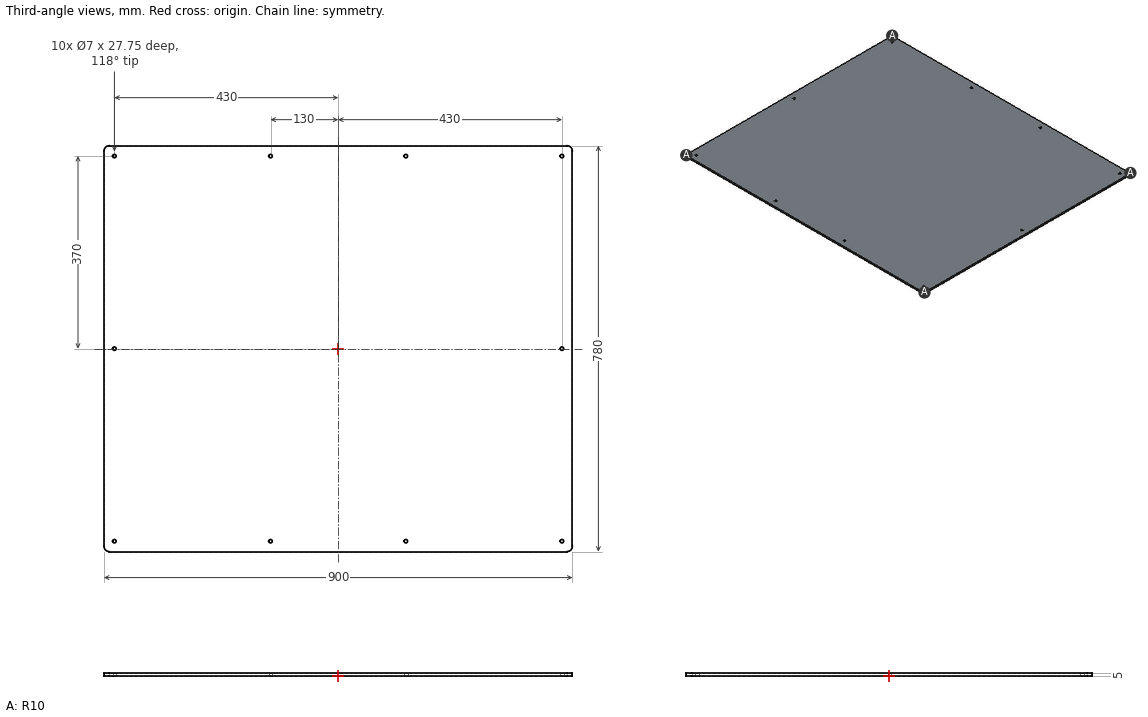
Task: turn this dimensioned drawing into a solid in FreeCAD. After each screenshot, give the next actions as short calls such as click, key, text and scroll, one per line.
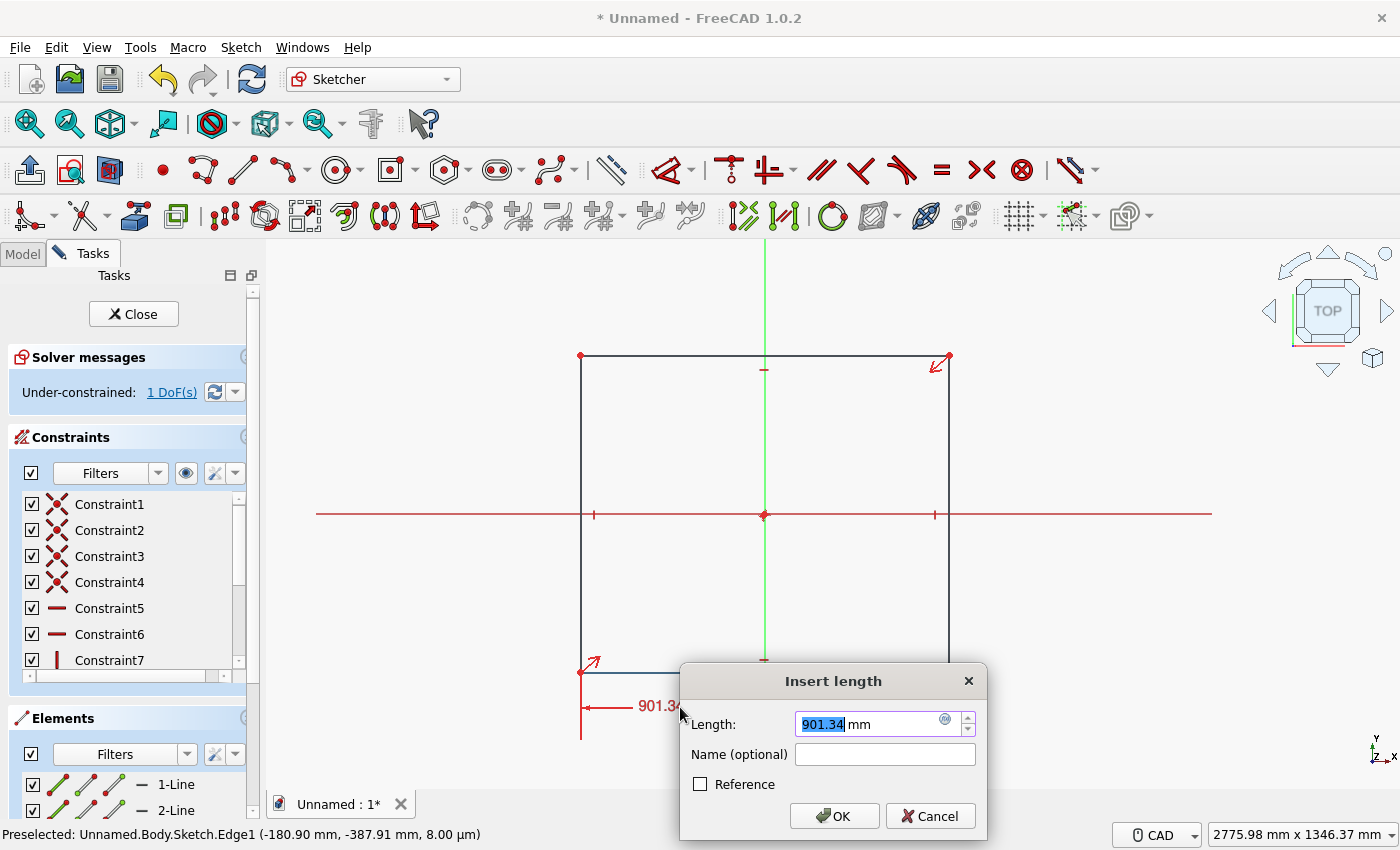
text(900)
key(Return)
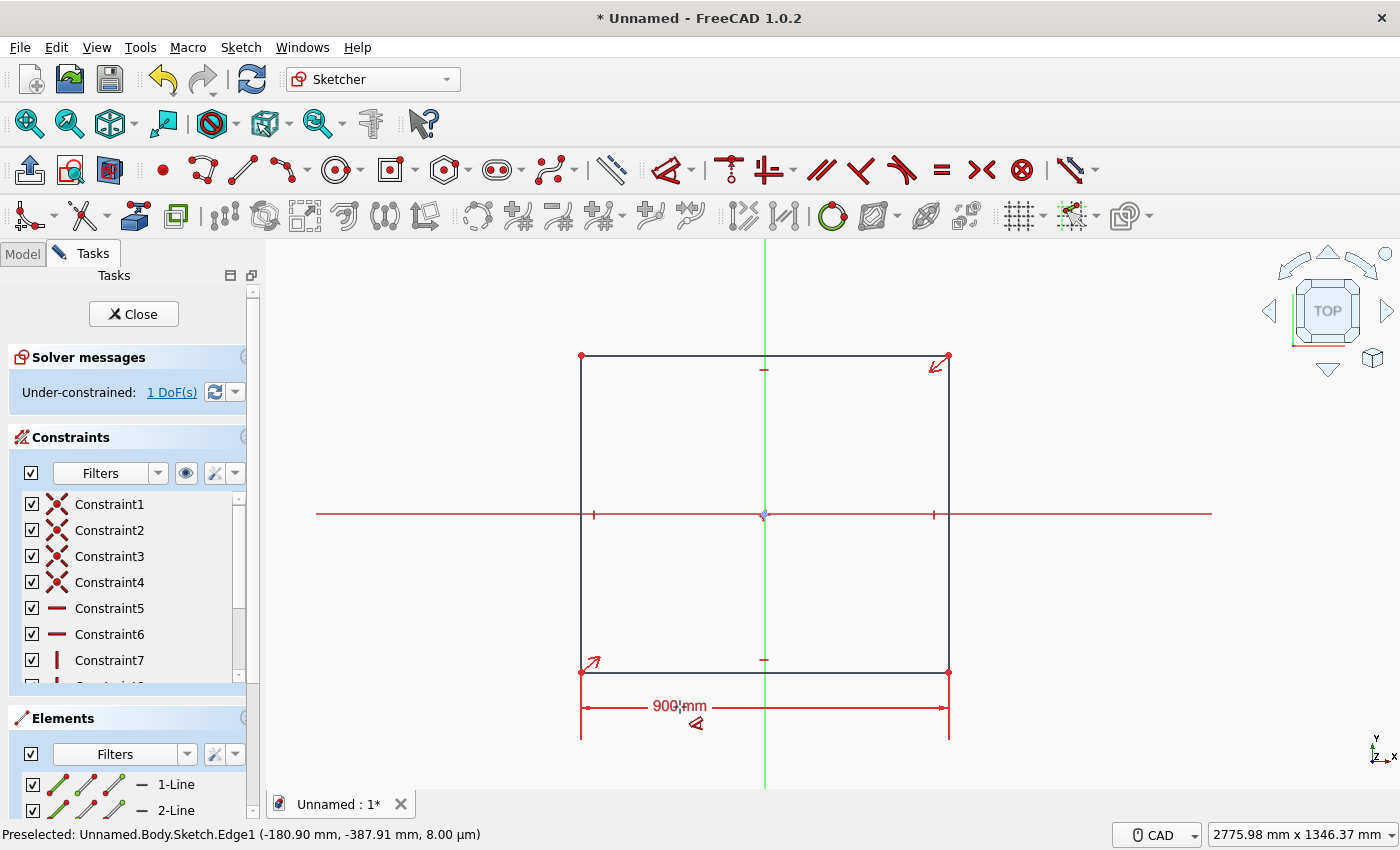
click(949, 578)
click(983, 442)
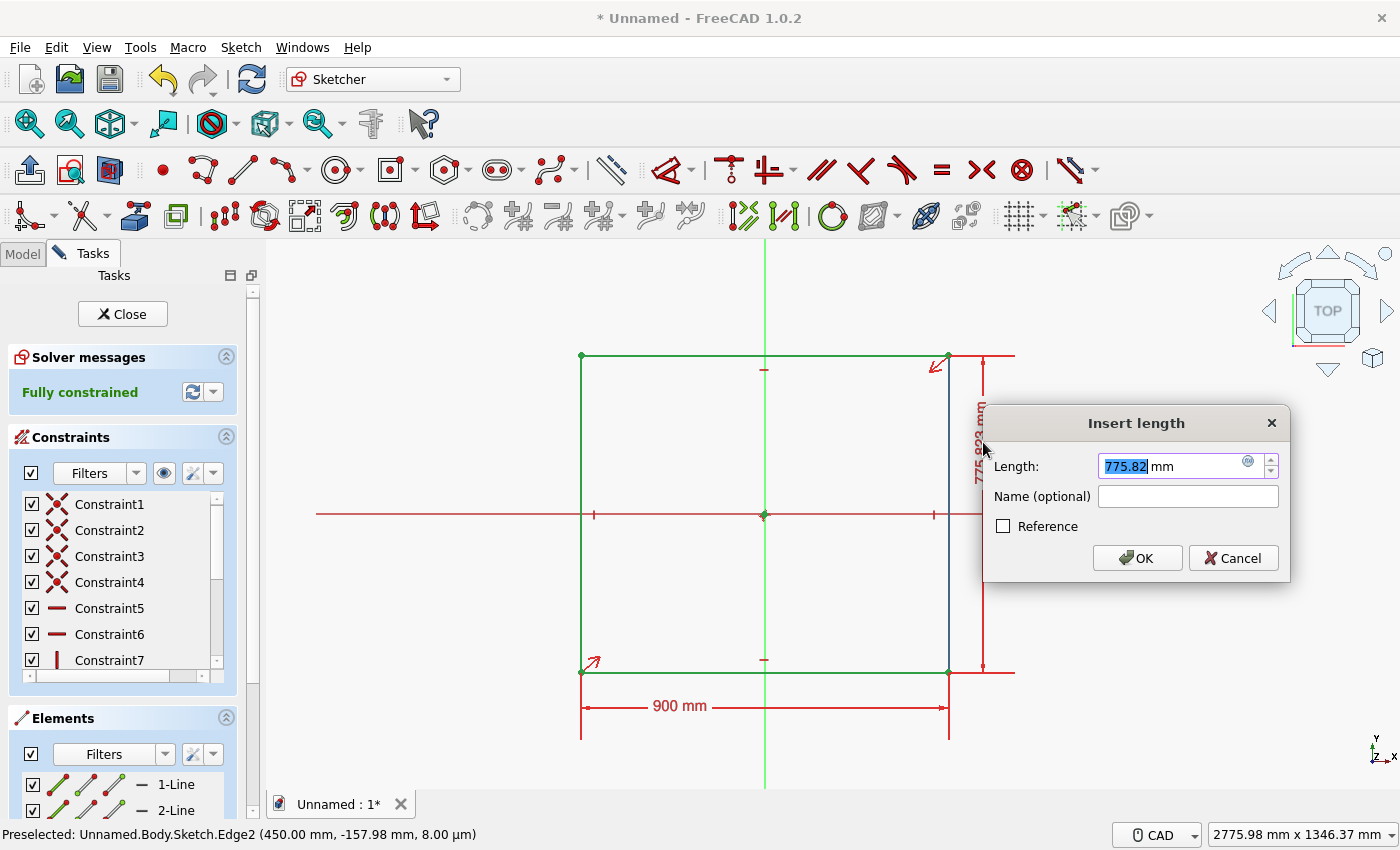
text(780)
key(Return)
key(Escape)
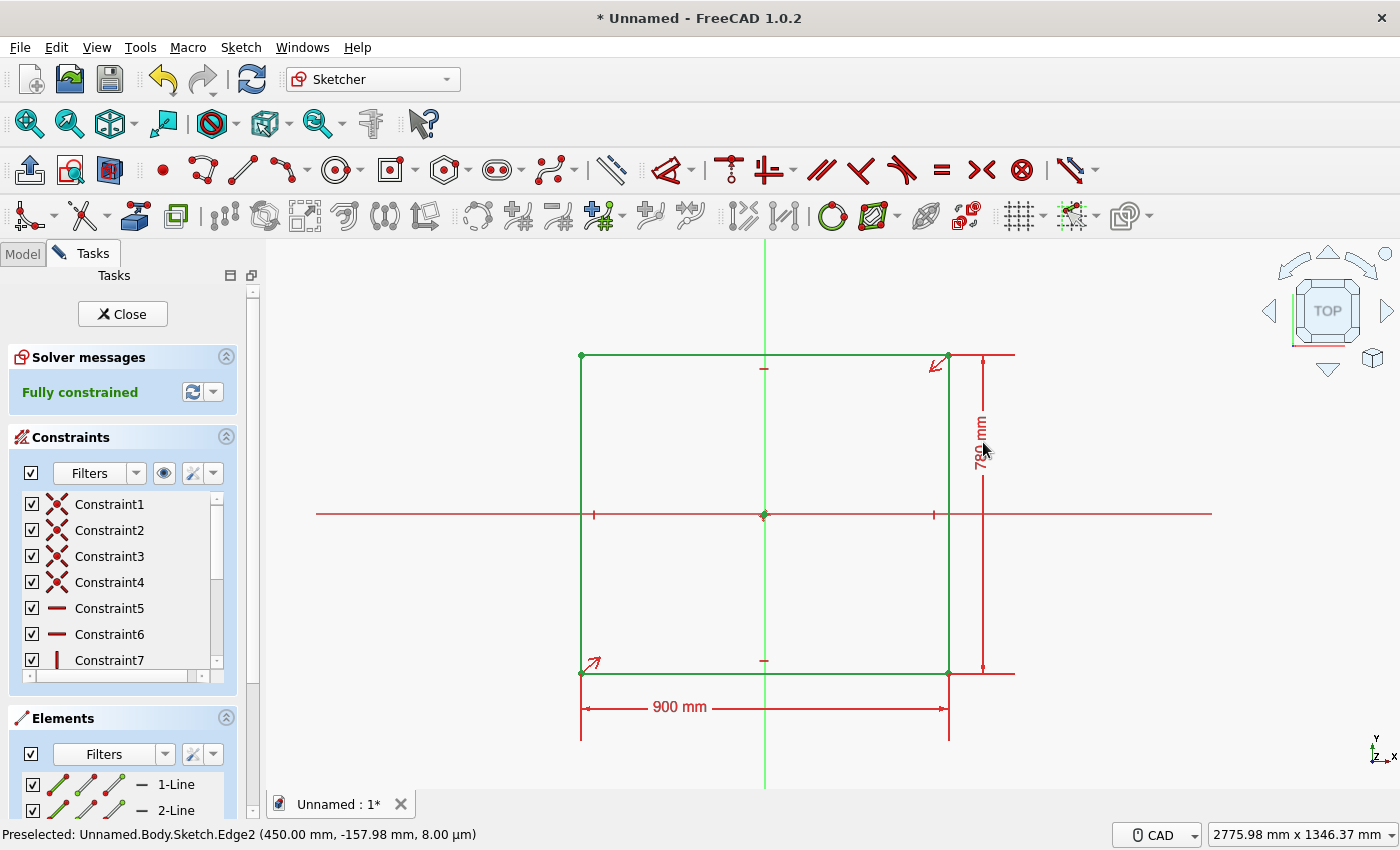
click(123, 314)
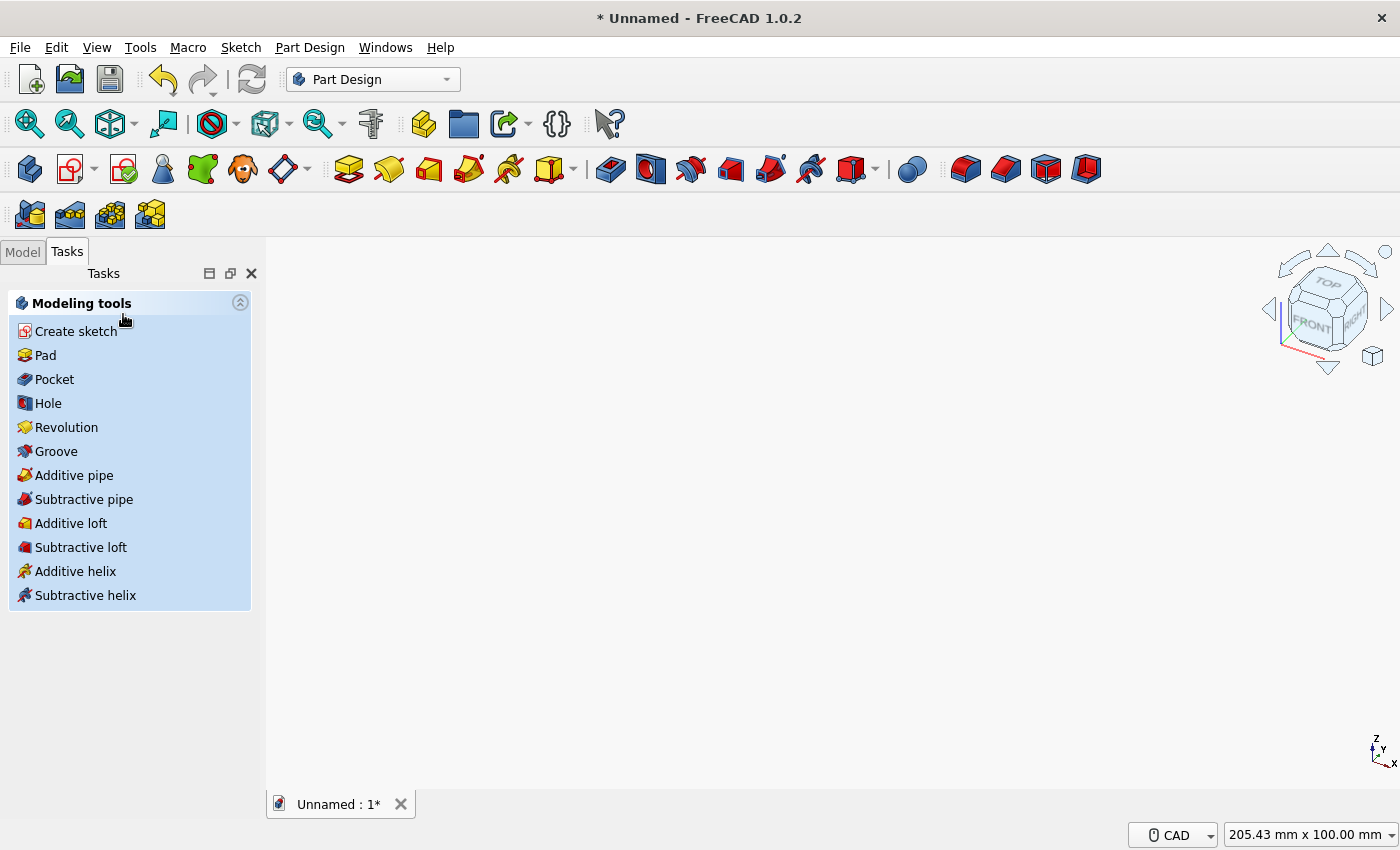
click(350, 170)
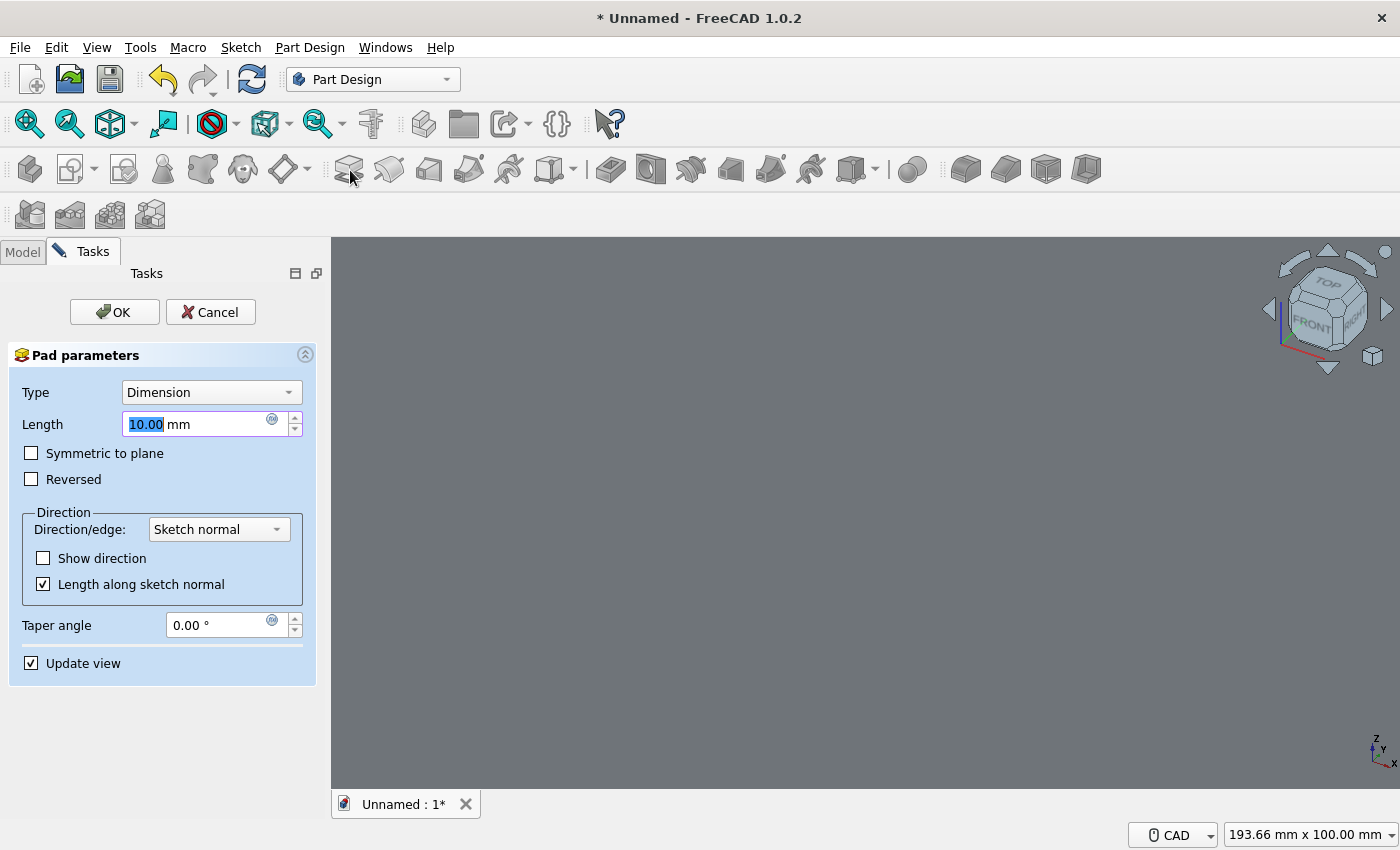
text(5)
key(Tab)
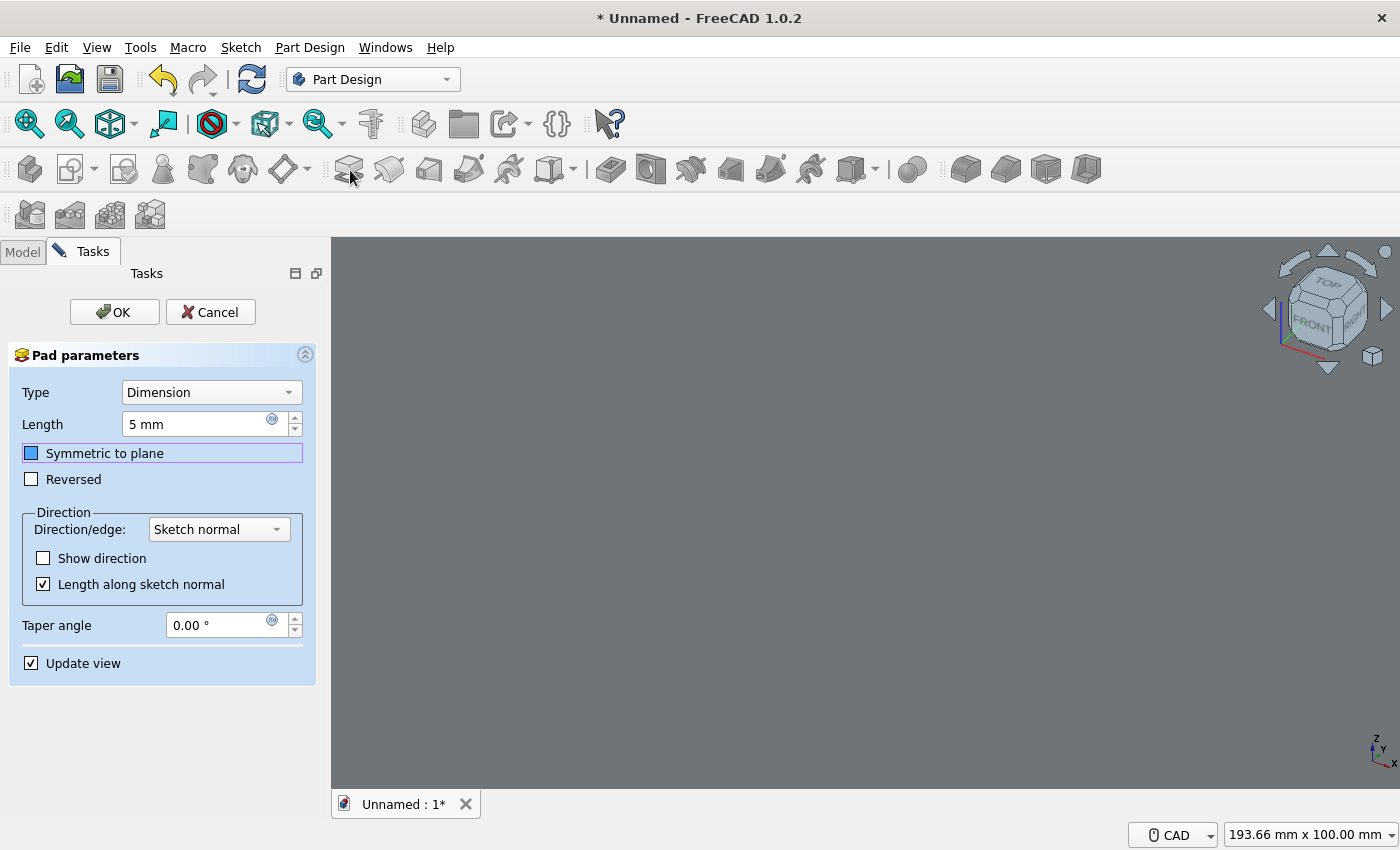
click(115, 312)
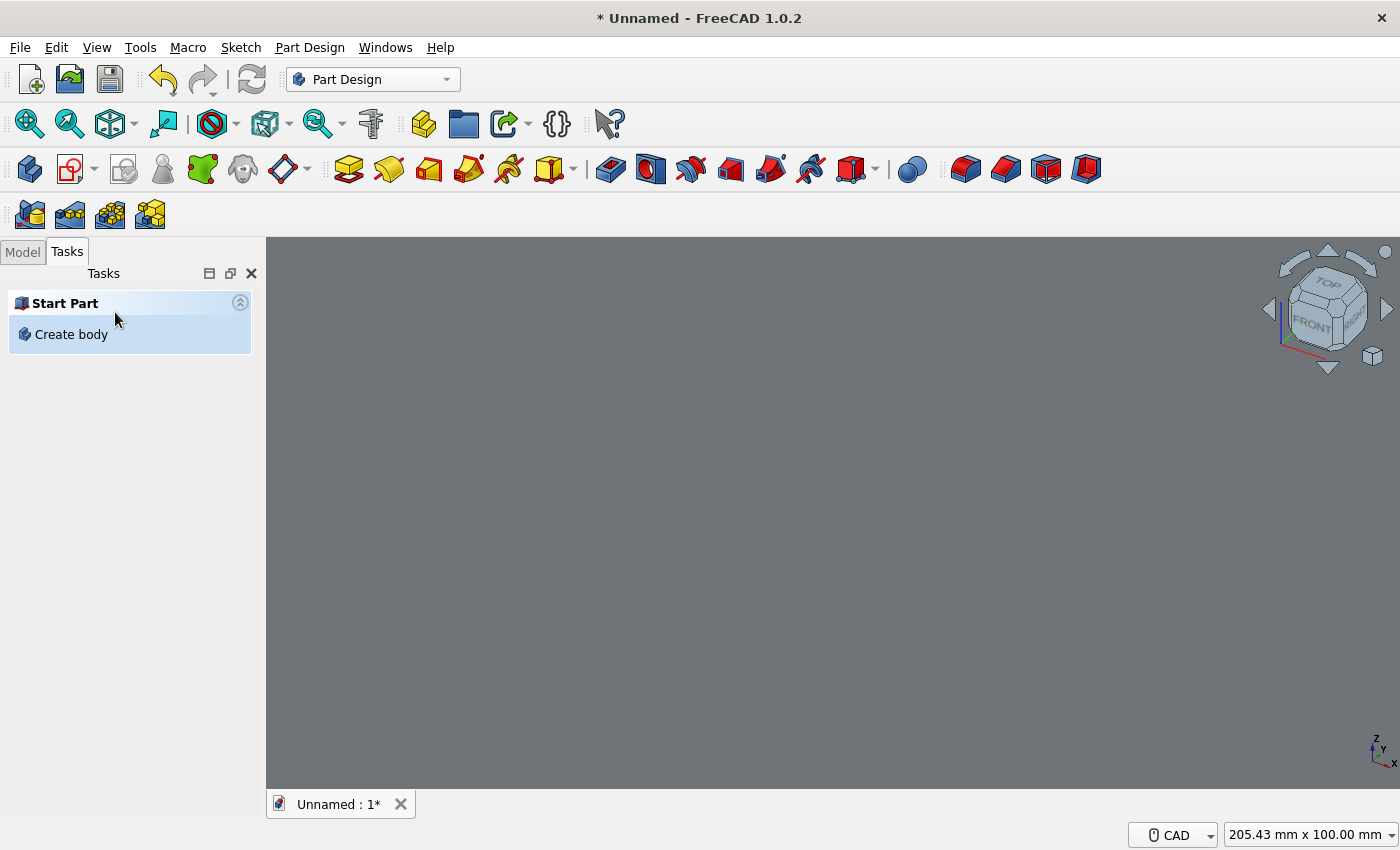
click(30, 124)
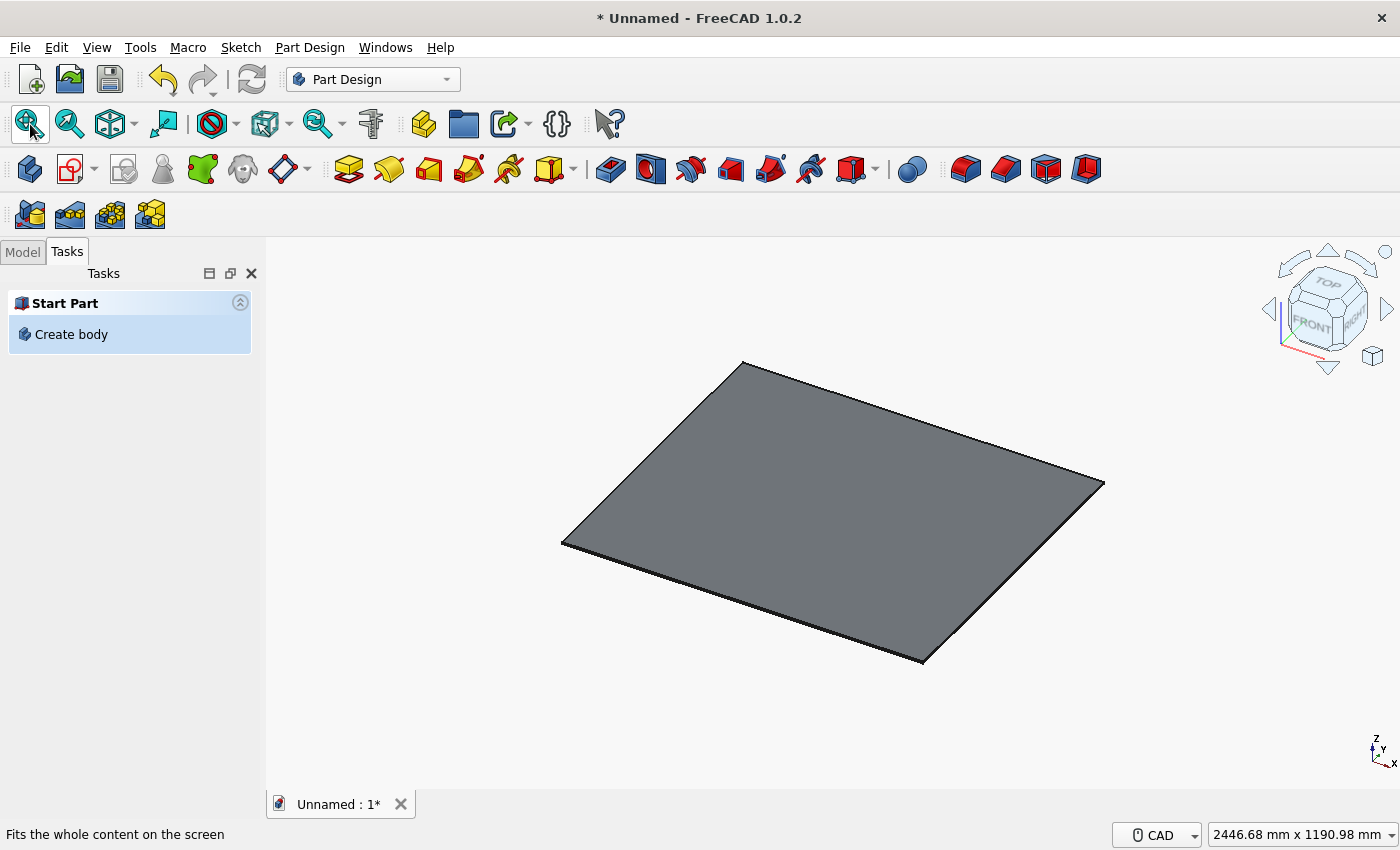
click(833, 511)